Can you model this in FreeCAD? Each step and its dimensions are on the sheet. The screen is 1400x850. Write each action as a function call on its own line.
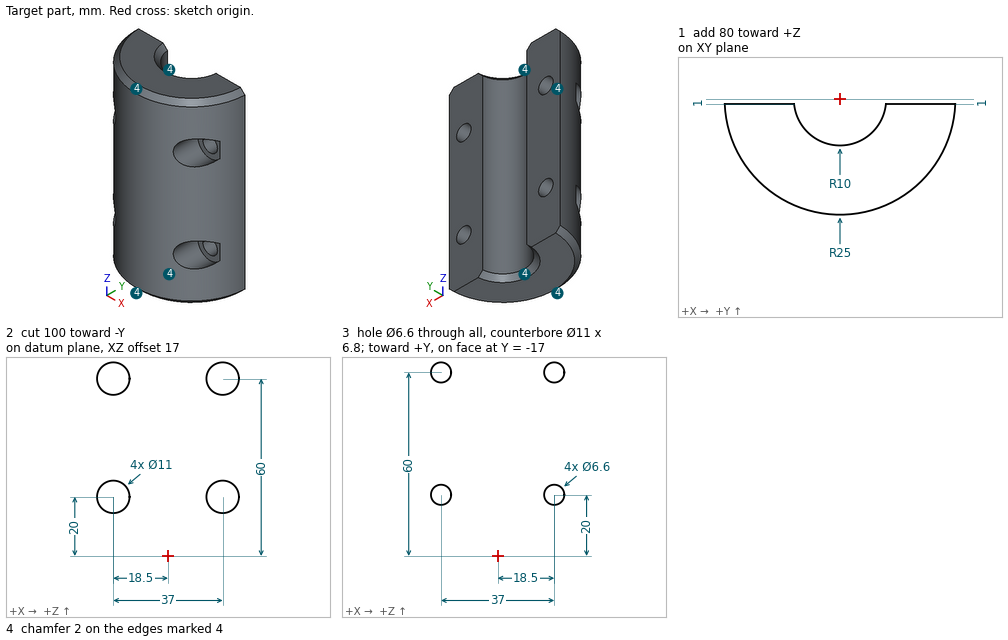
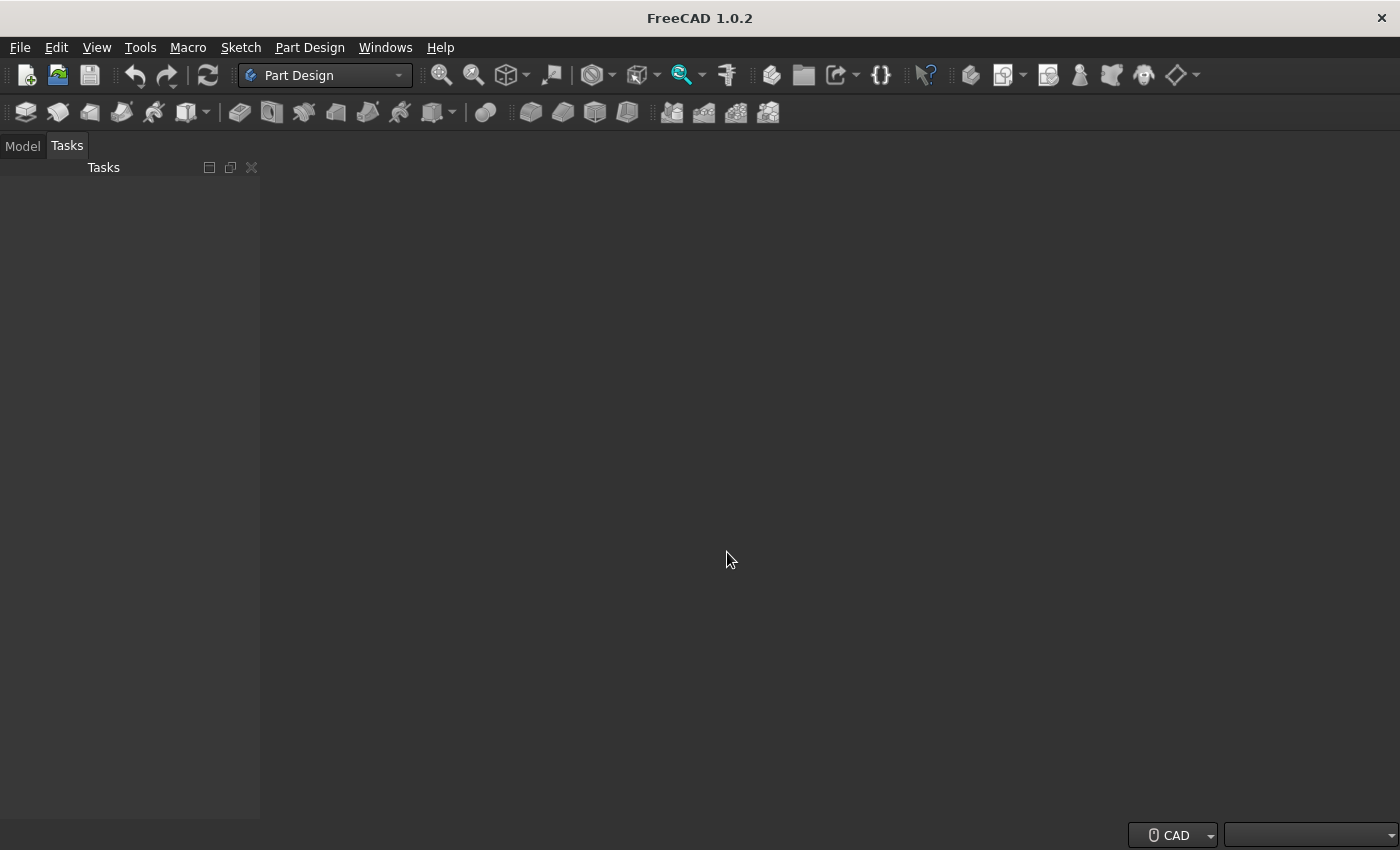
click(26, 76)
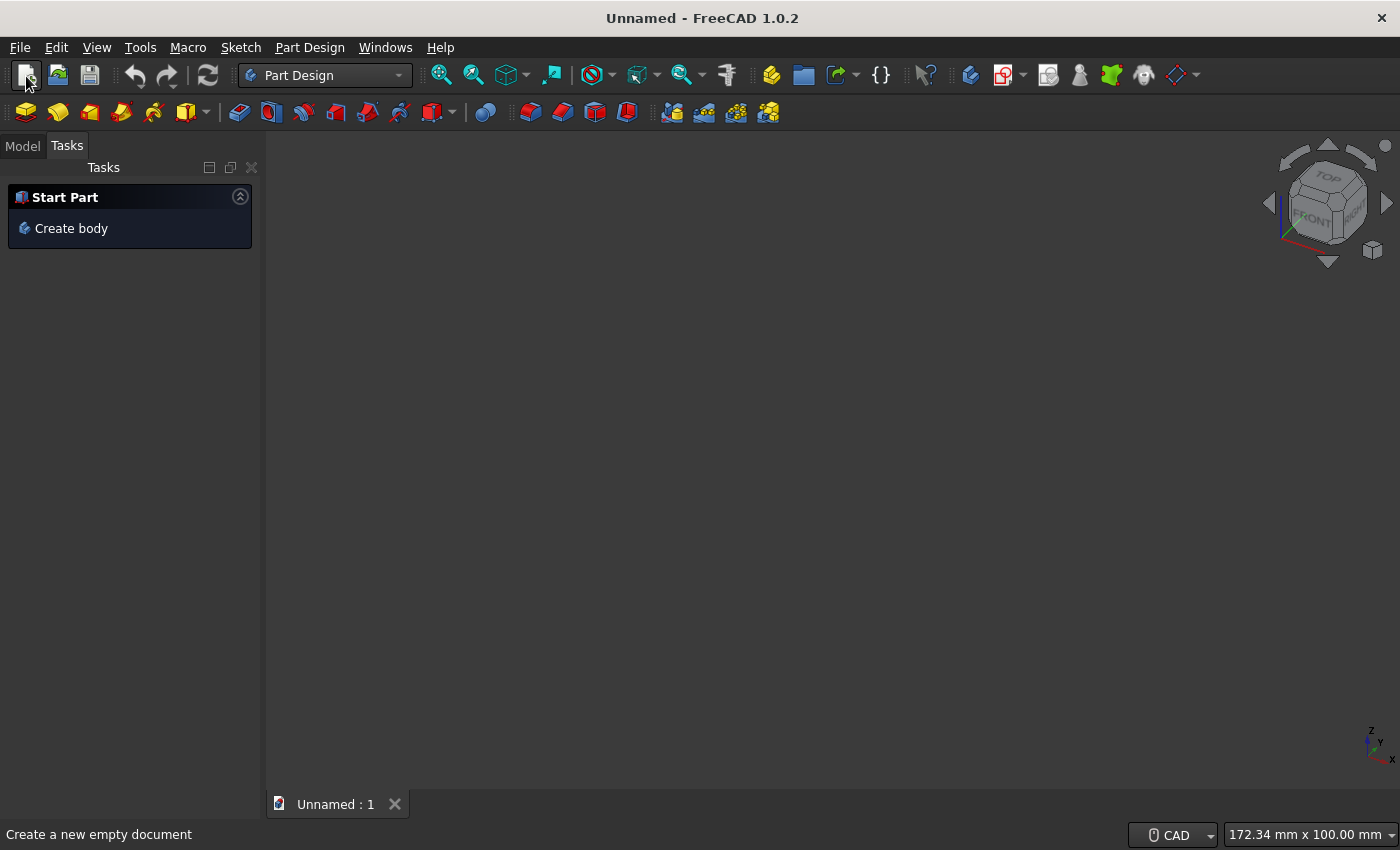
click(1004, 76)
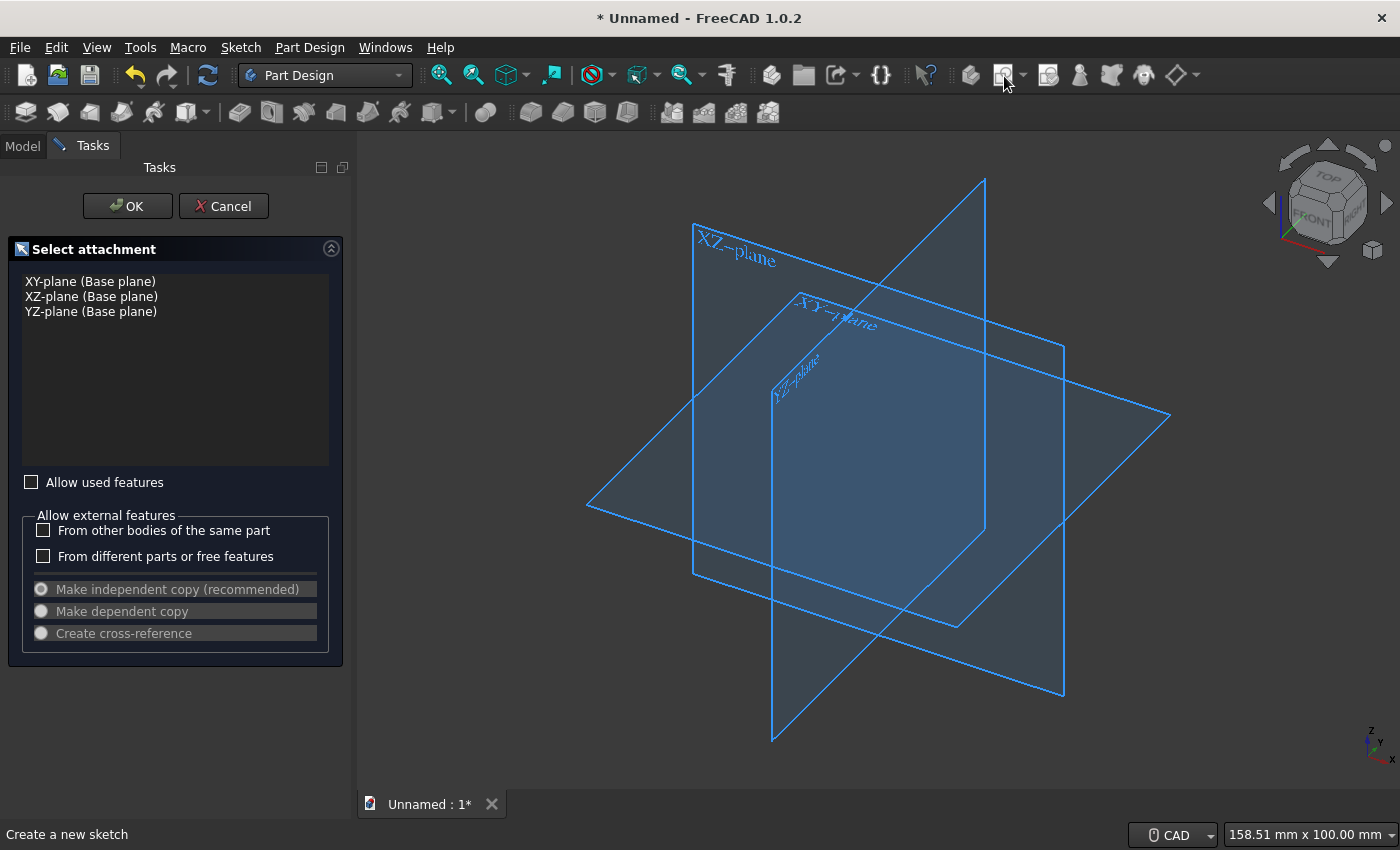
click(82, 282)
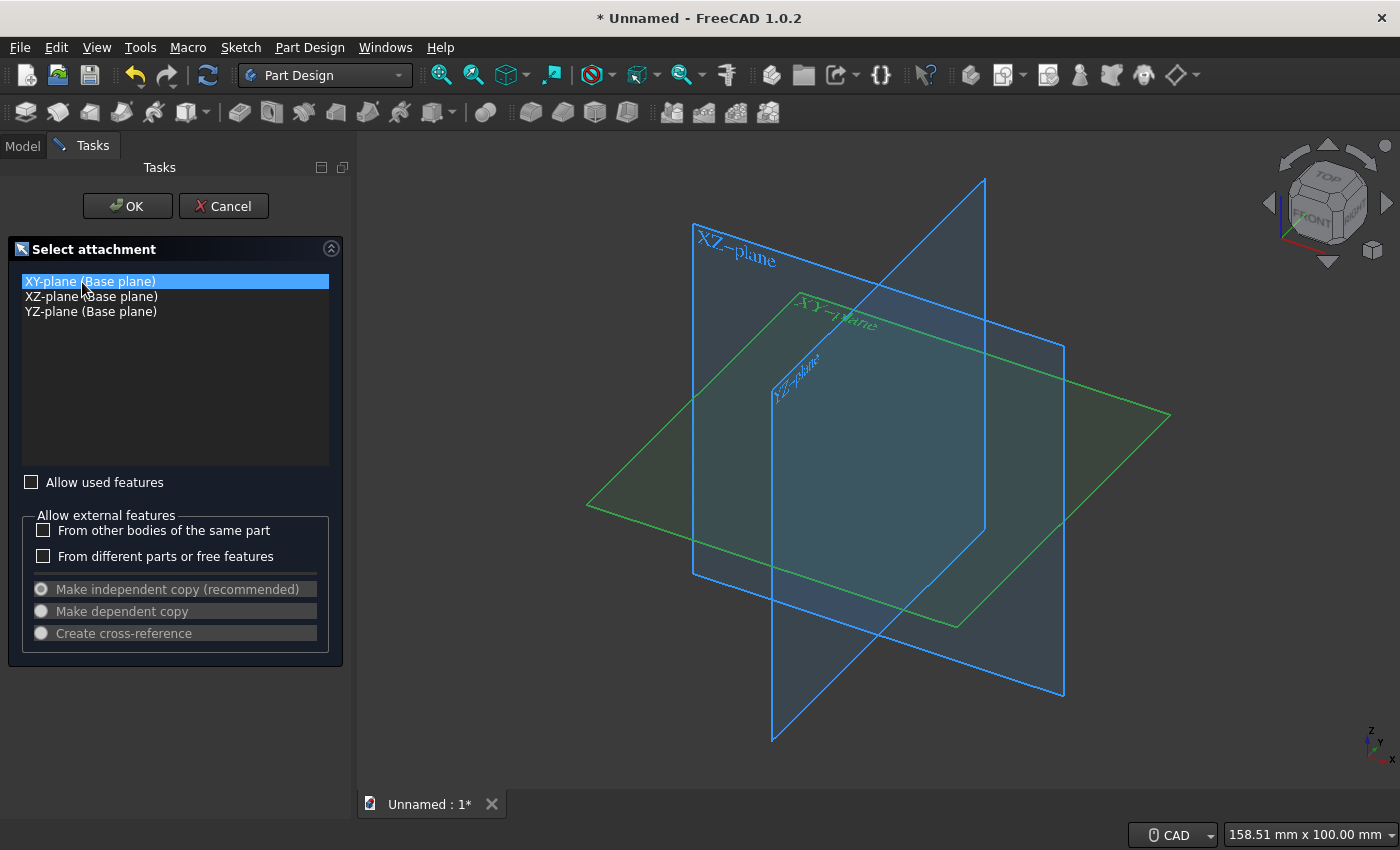
click(128, 206)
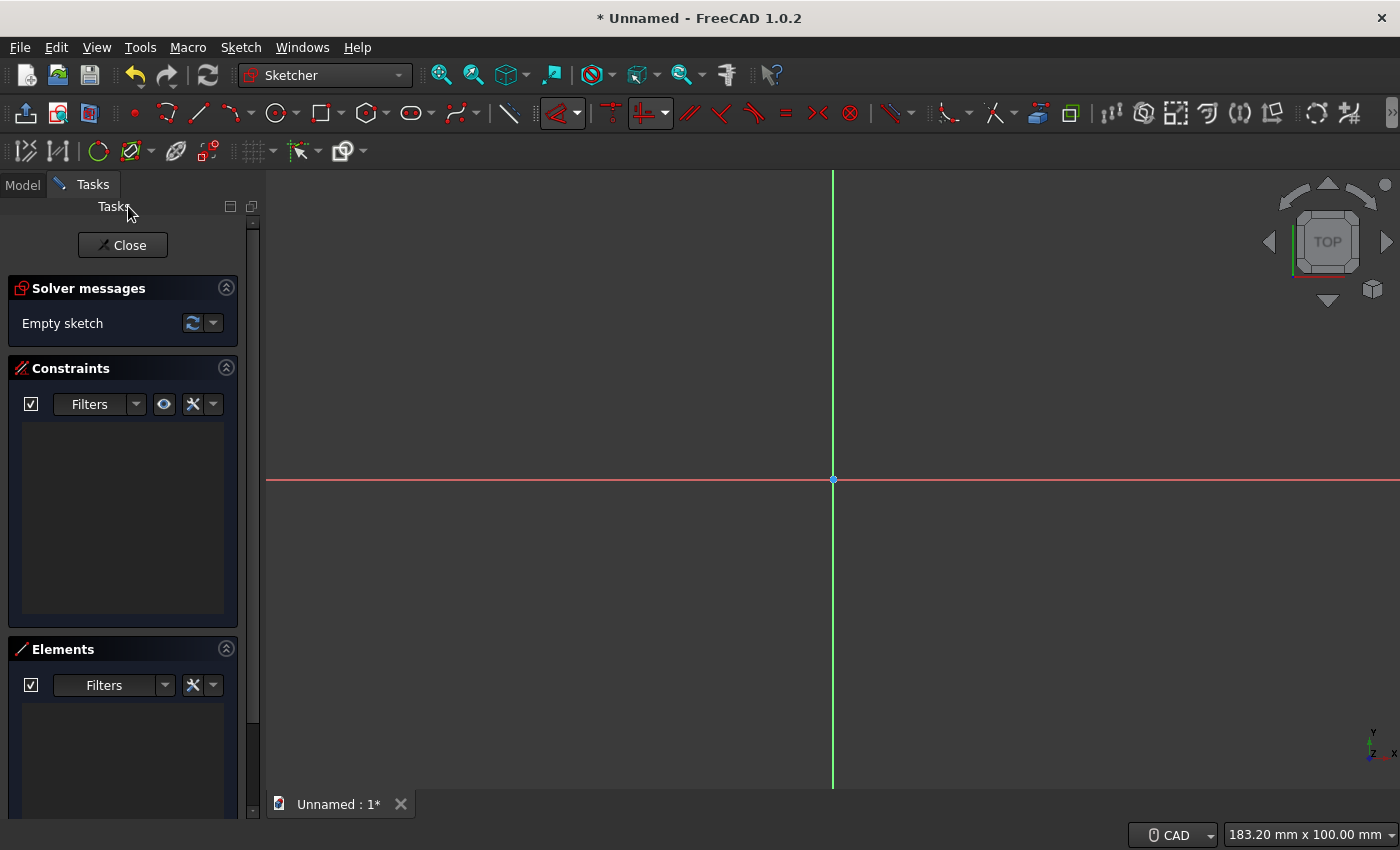
scroll(889, 620, up, 4)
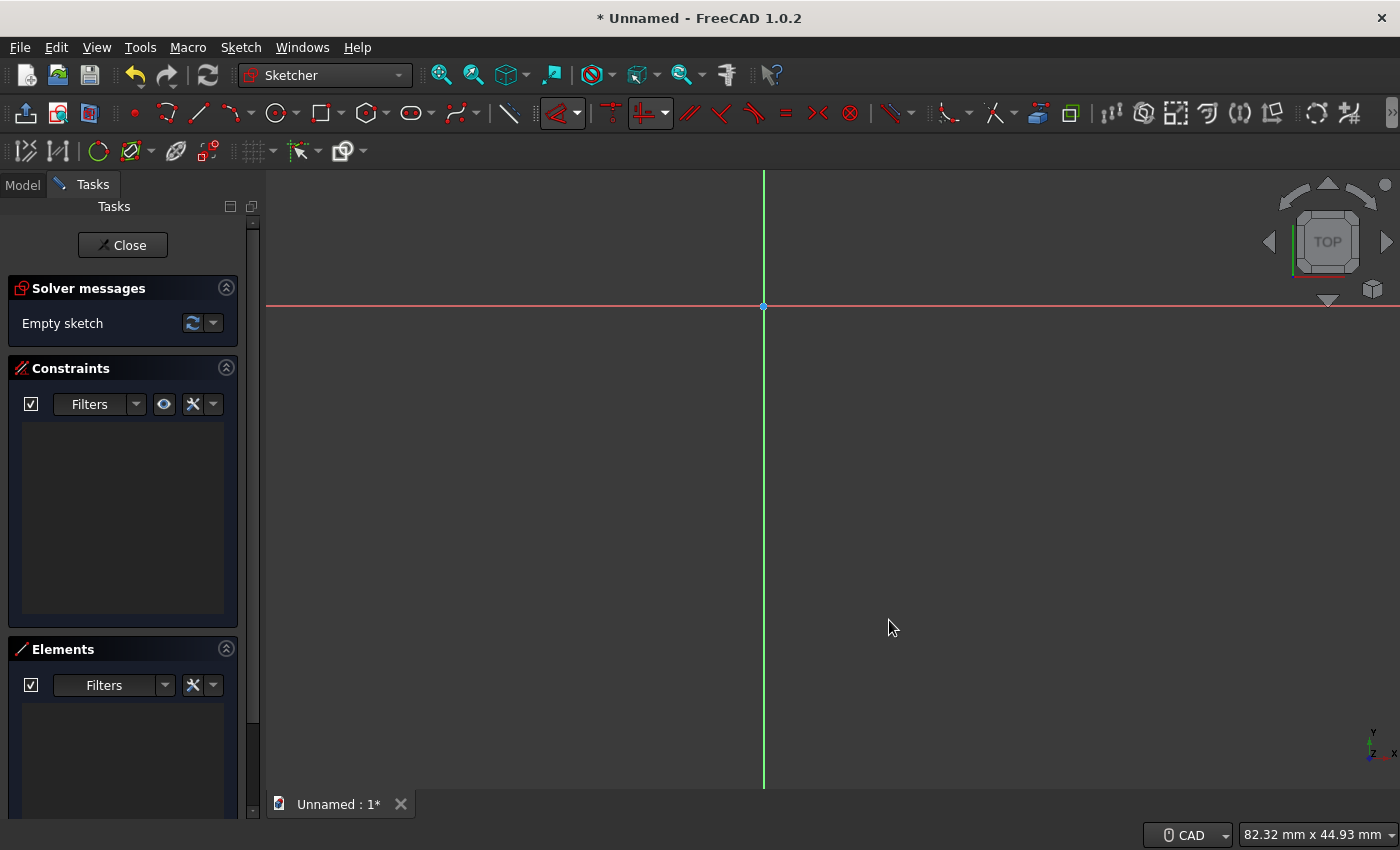
click(200, 114)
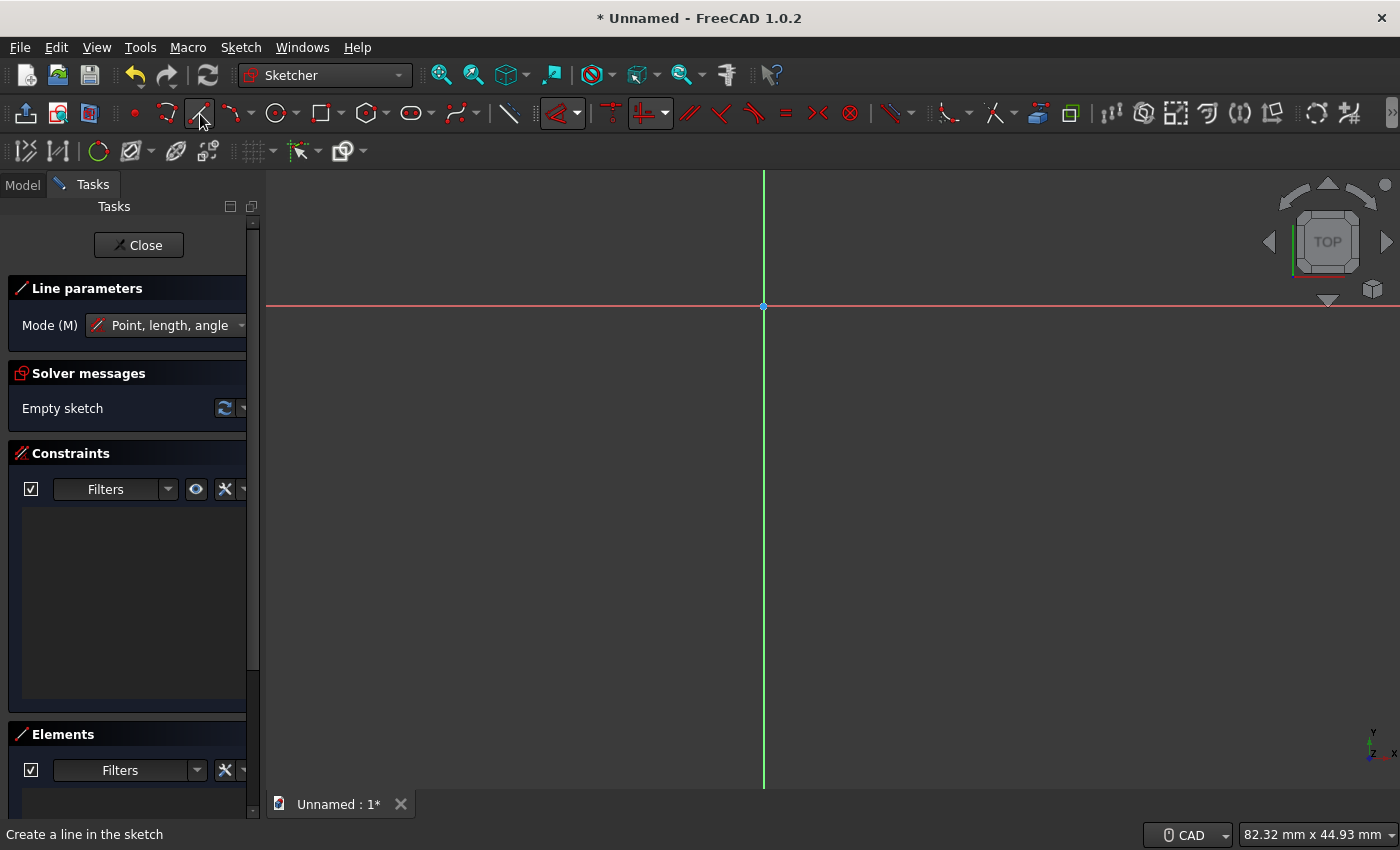
click(627, 320)
click(420, 320)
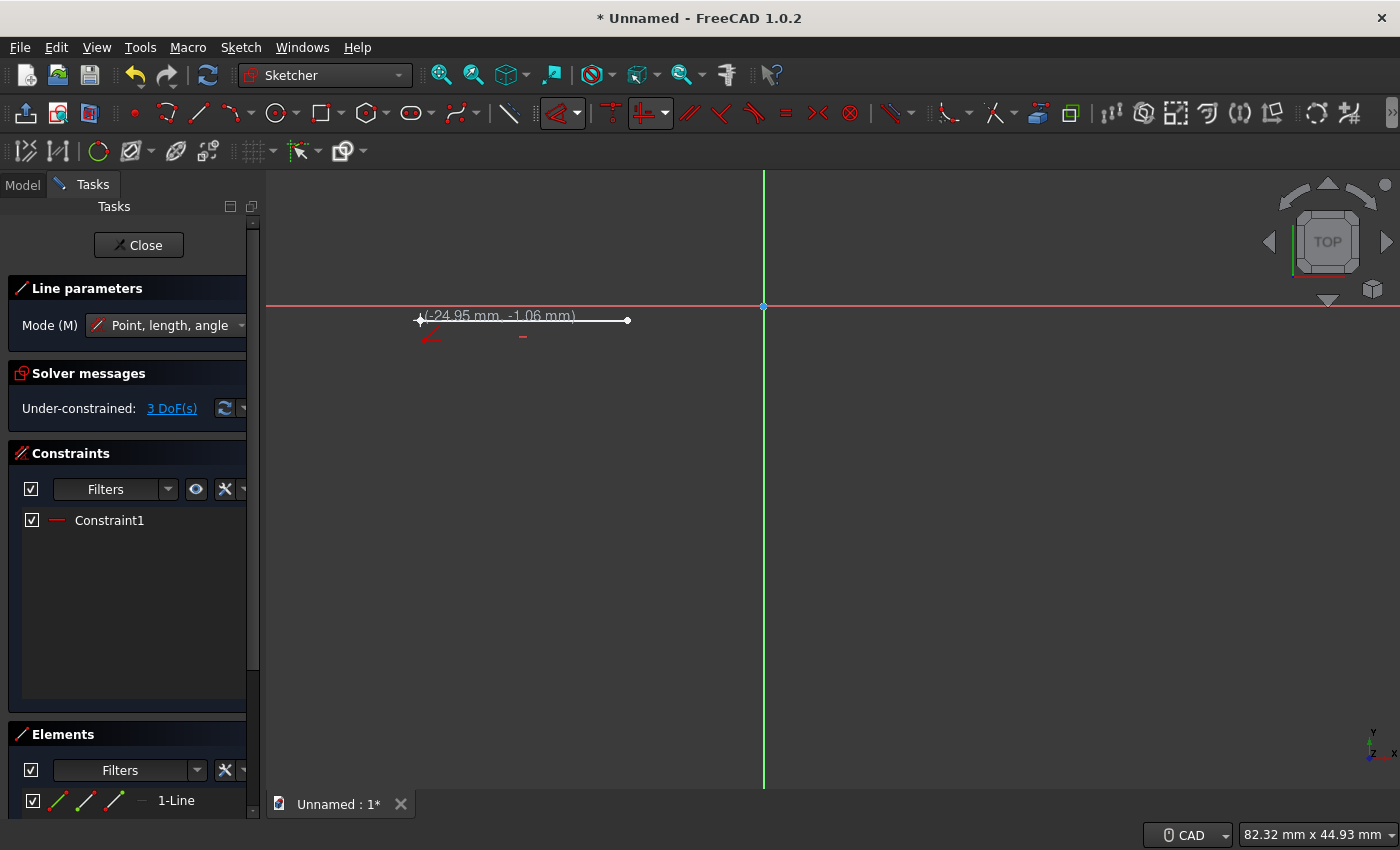
click(1108, 320)
click(901, 320)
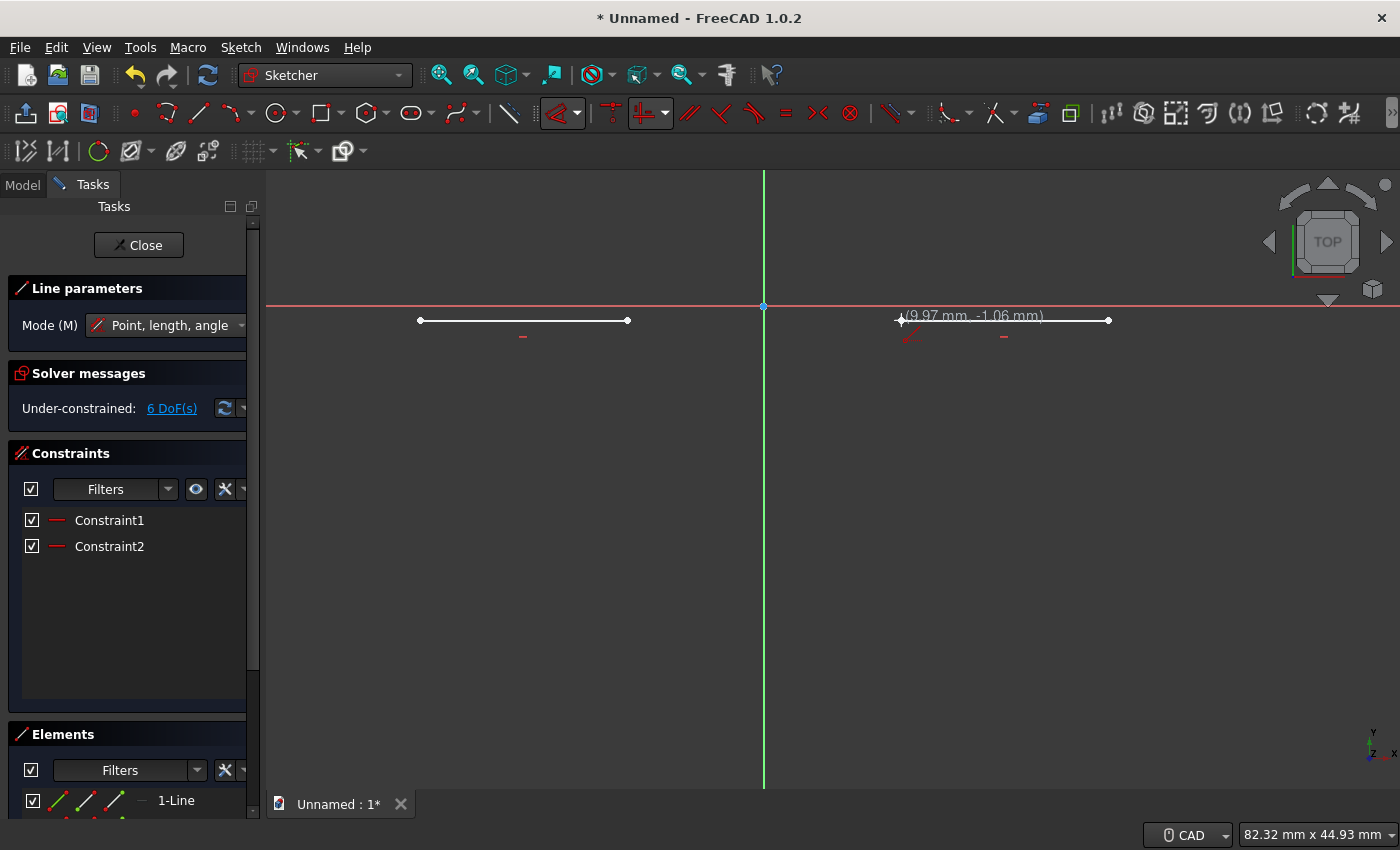
click(232, 114)